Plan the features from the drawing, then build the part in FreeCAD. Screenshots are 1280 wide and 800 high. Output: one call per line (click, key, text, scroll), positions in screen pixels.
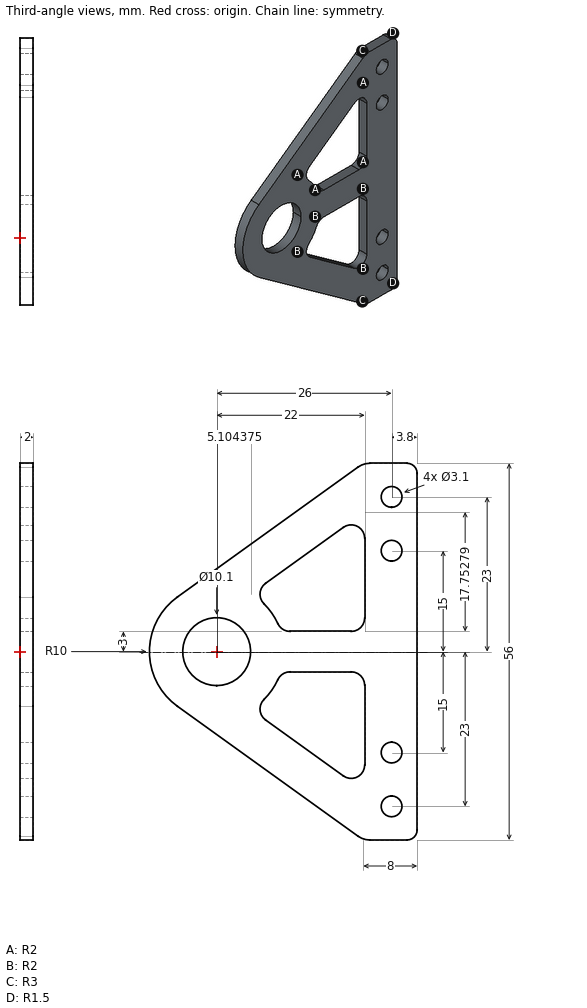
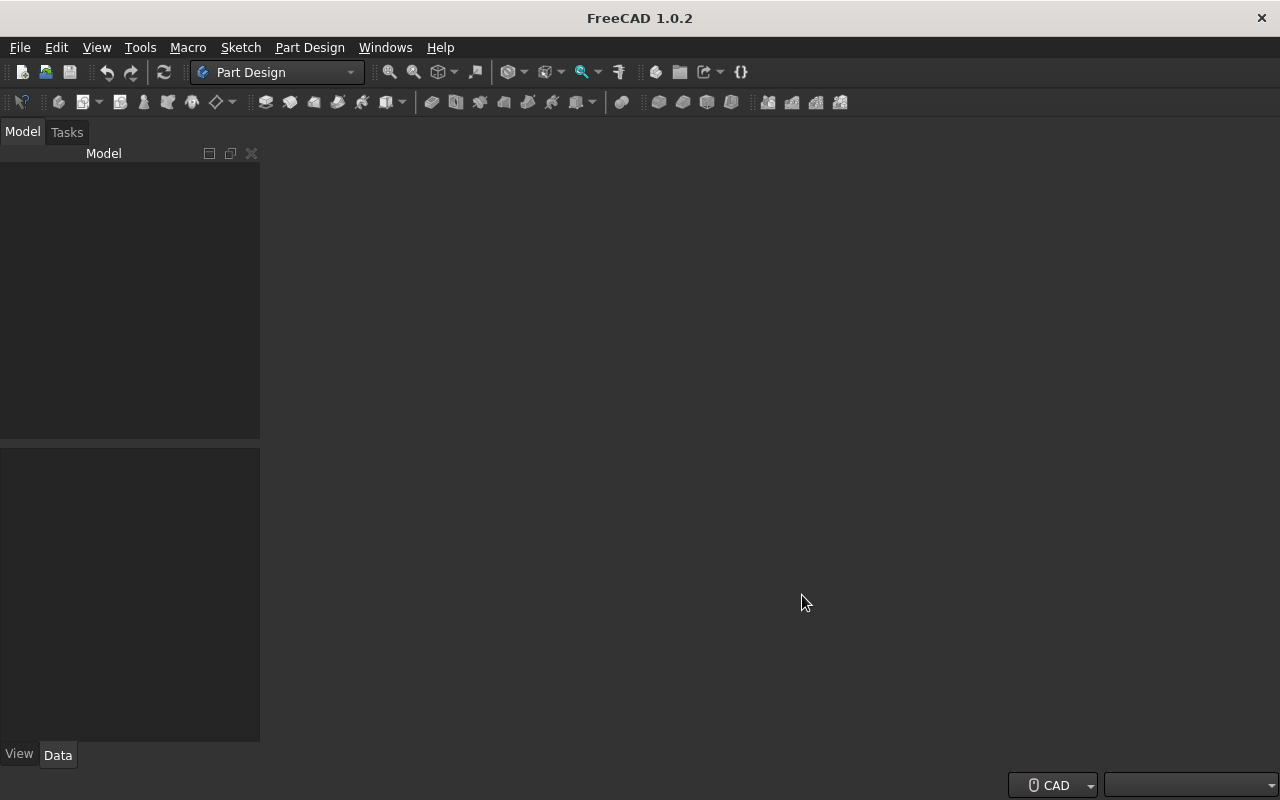
click(22, 72)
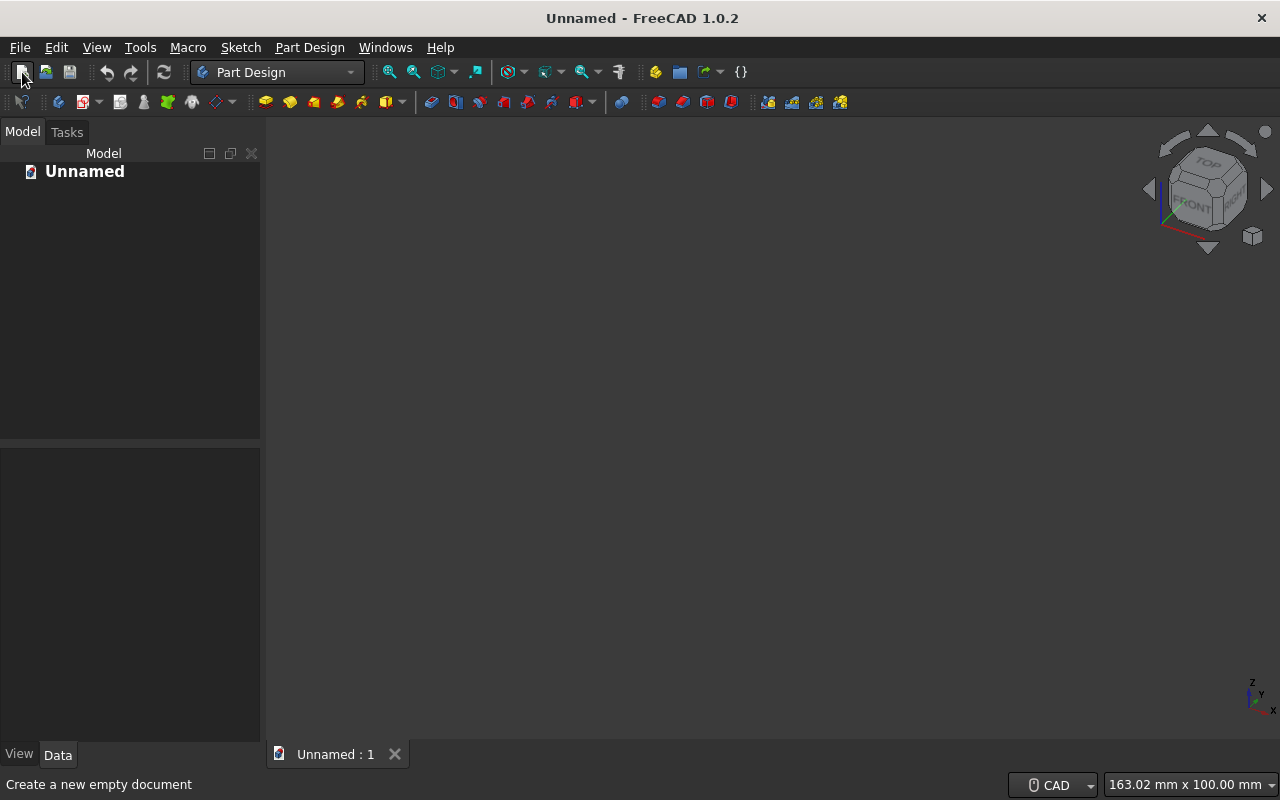
click(84, 102)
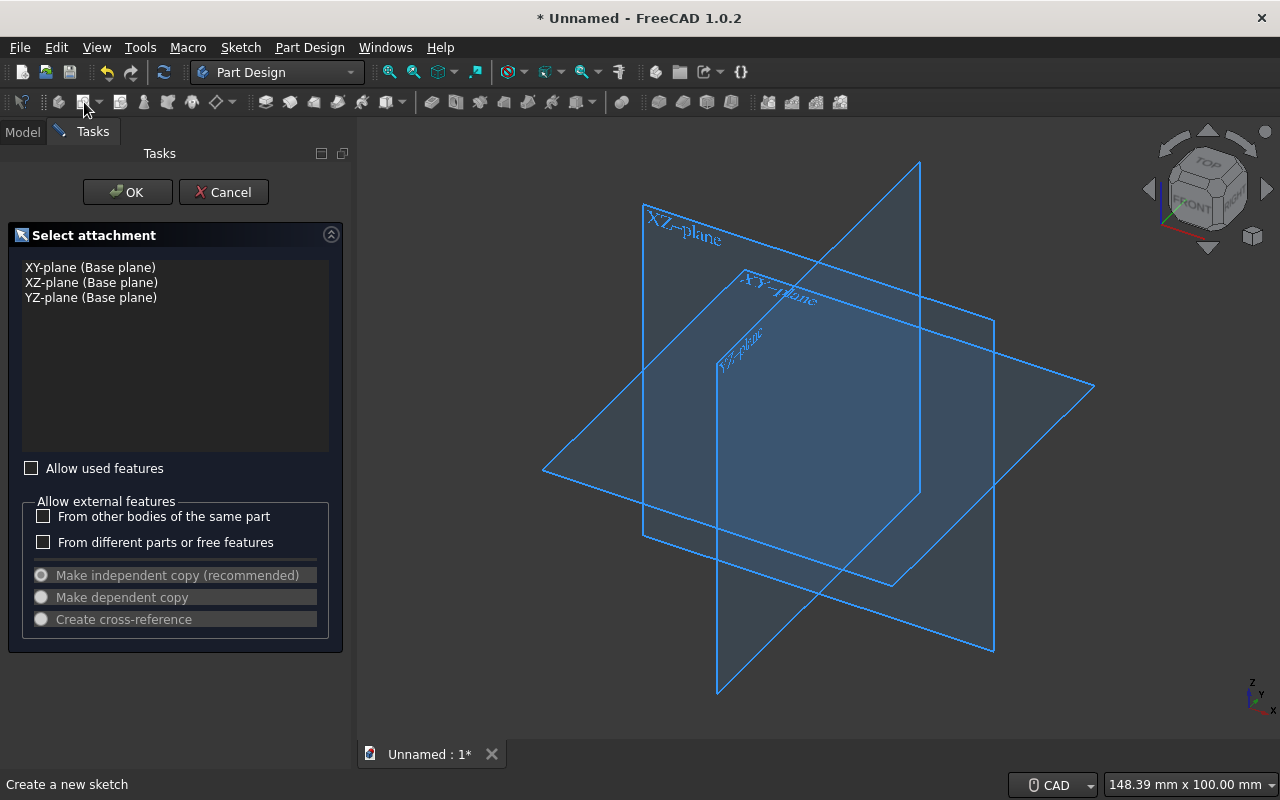
click(82, 298)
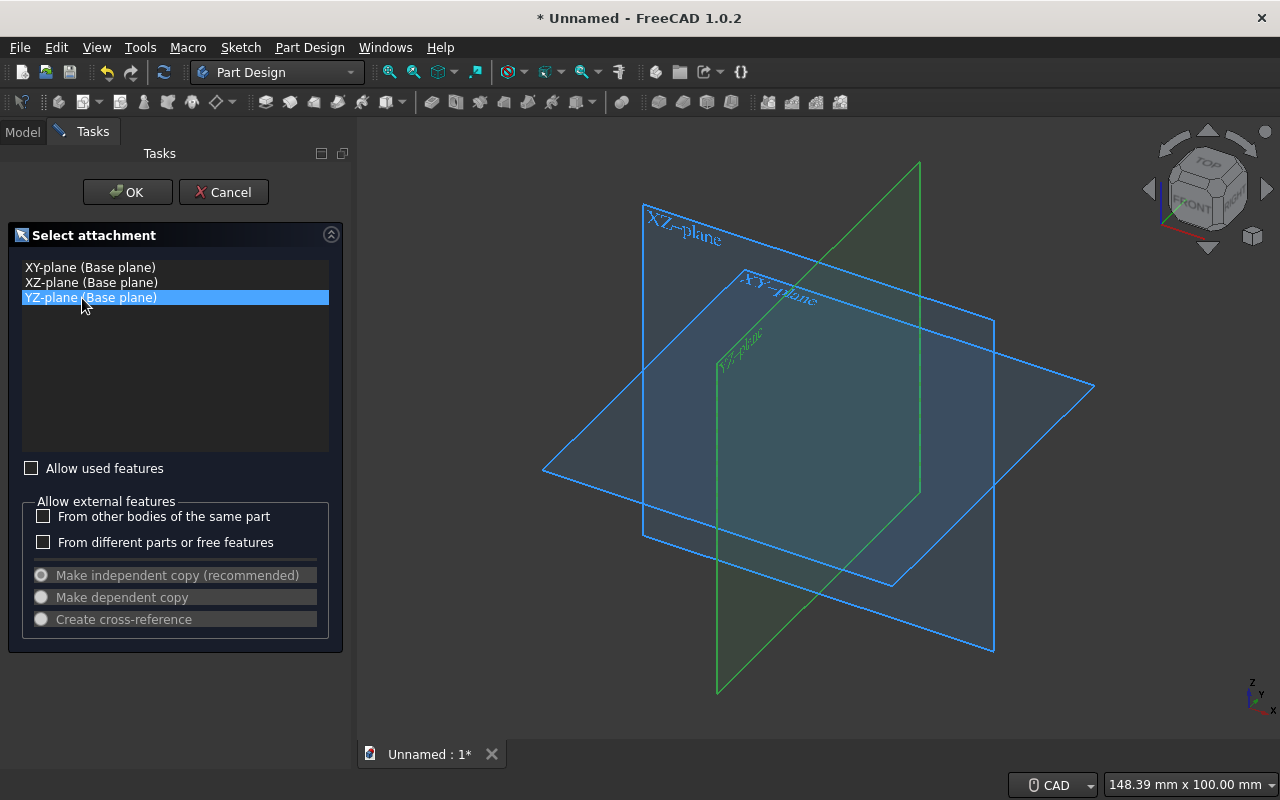
click(128, 192)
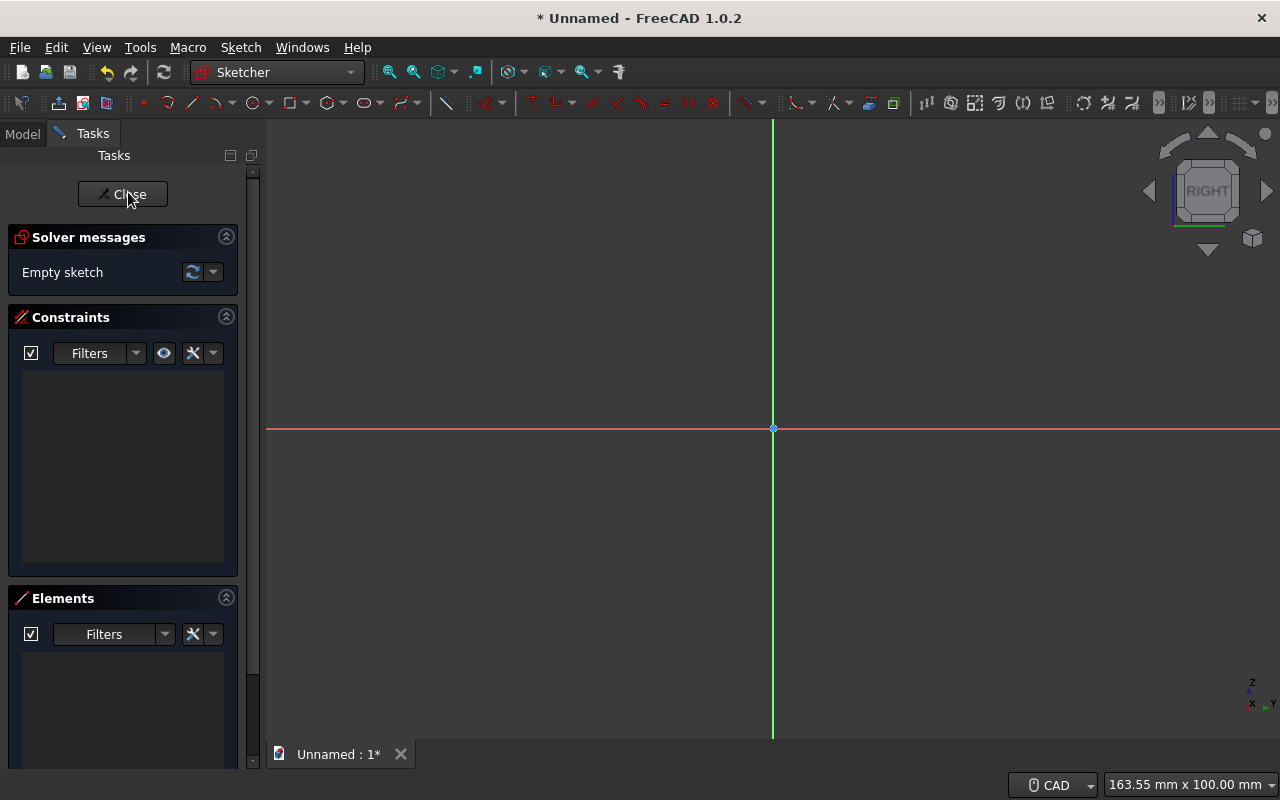
click(168, 104)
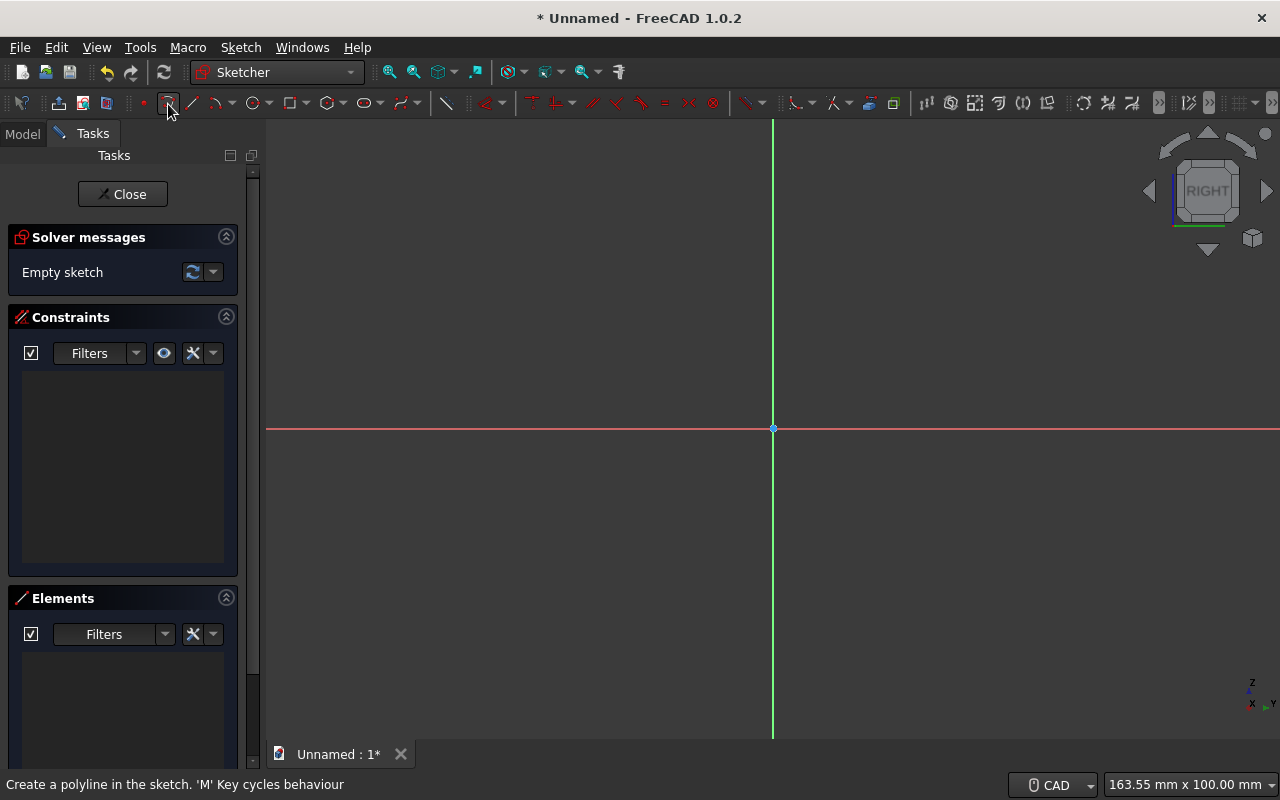
click(737, 479)
click(908, 603)
click(958, 603)
click(958, 255)
click(908, 255)
click(737, 379)
right_click(737, 379)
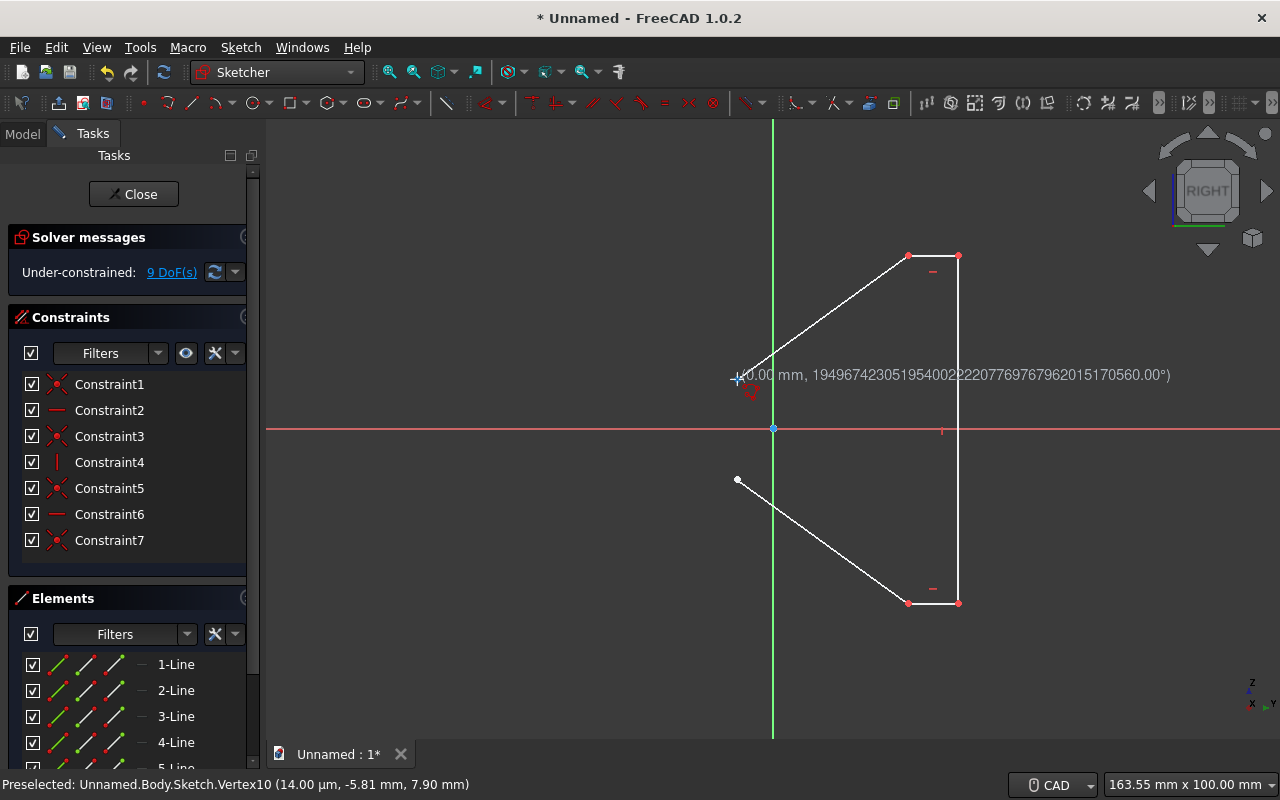
key(g)
key(3)
key(a)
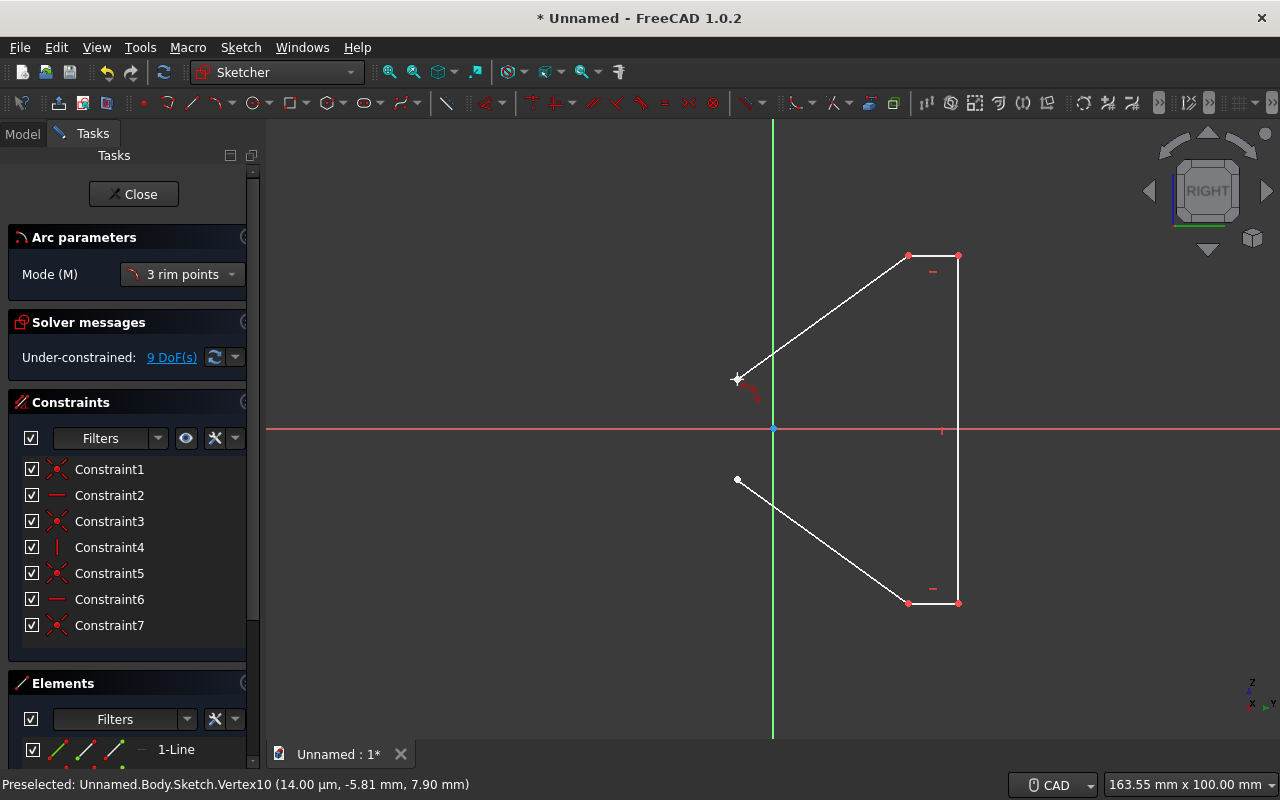
click(737, 380)
click(737, 480)
click(715, 406)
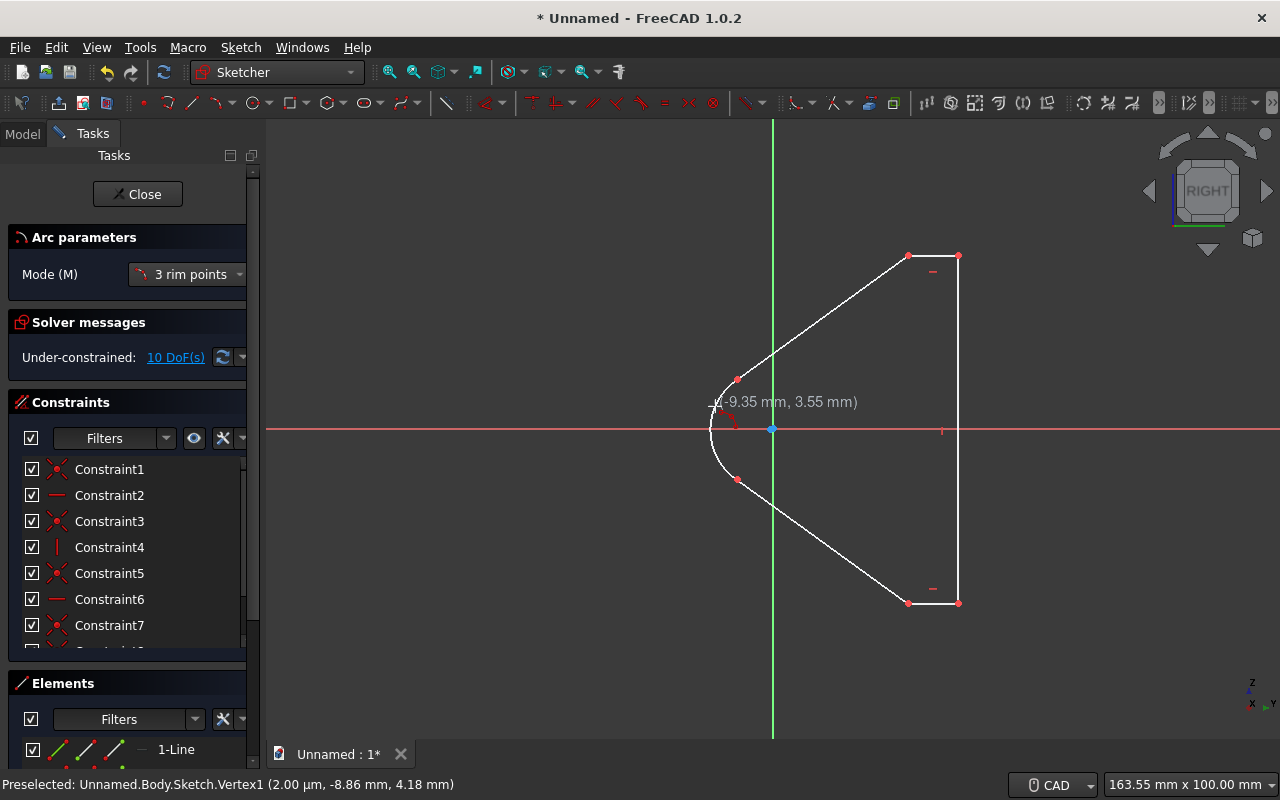
click(254, 104)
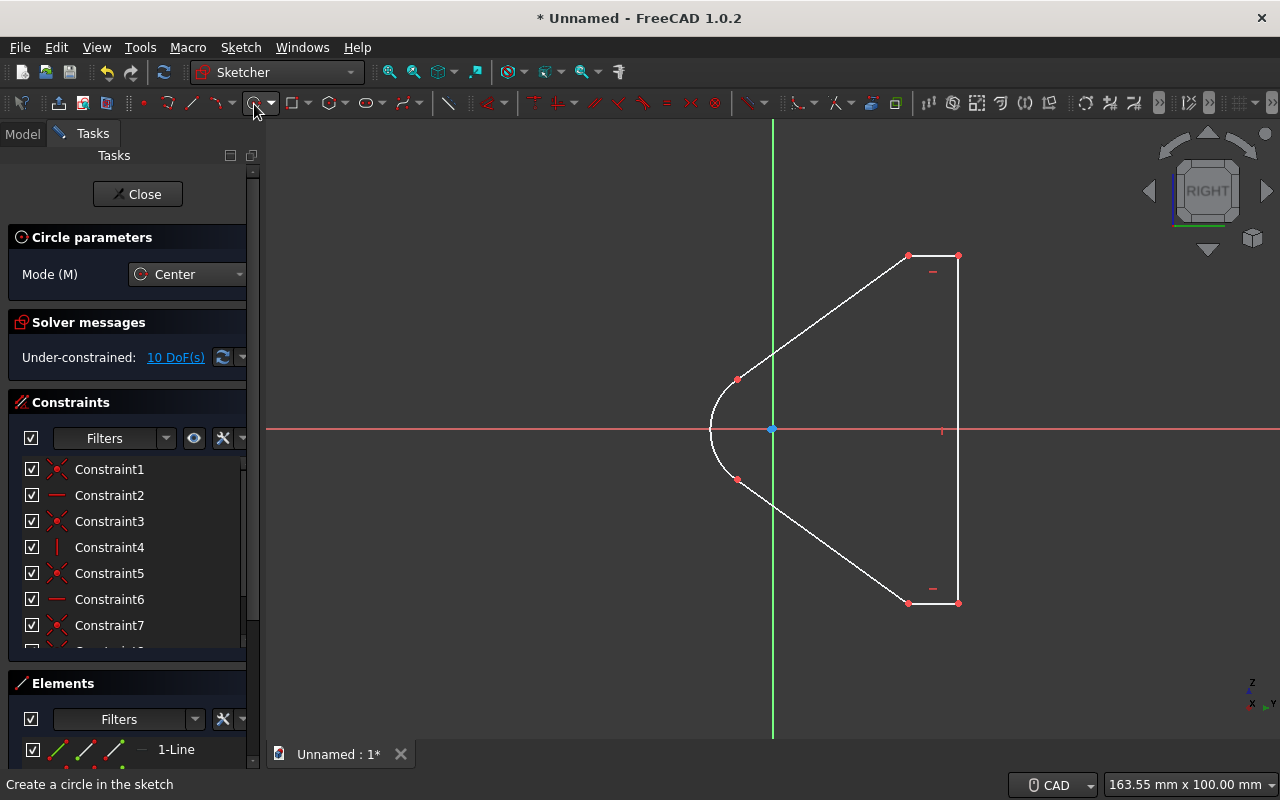
click(773, 429)
click(795, 407)